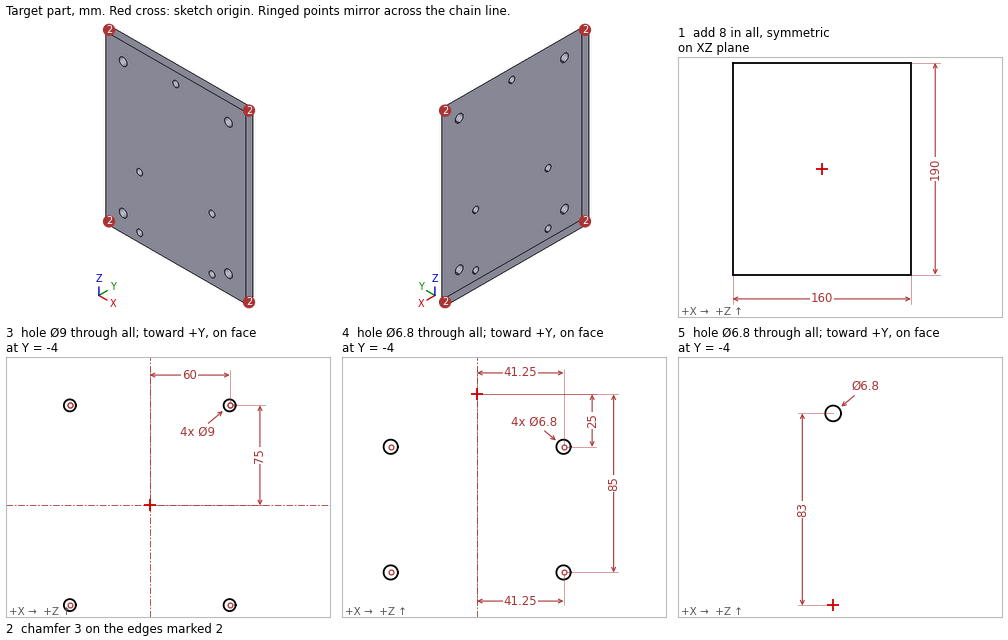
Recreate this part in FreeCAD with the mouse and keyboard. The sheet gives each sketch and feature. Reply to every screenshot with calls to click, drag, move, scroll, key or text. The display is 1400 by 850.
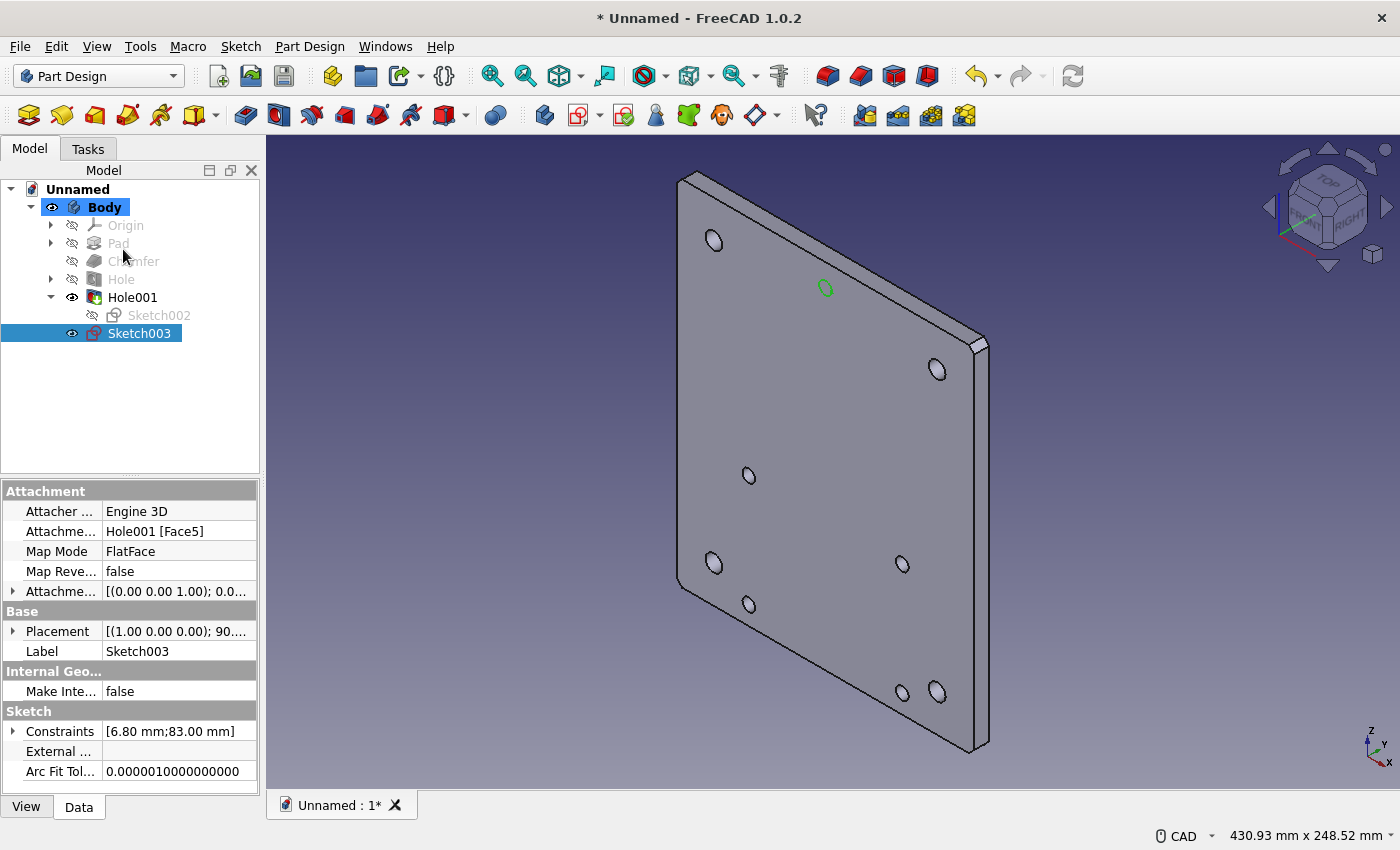
click(279, 116)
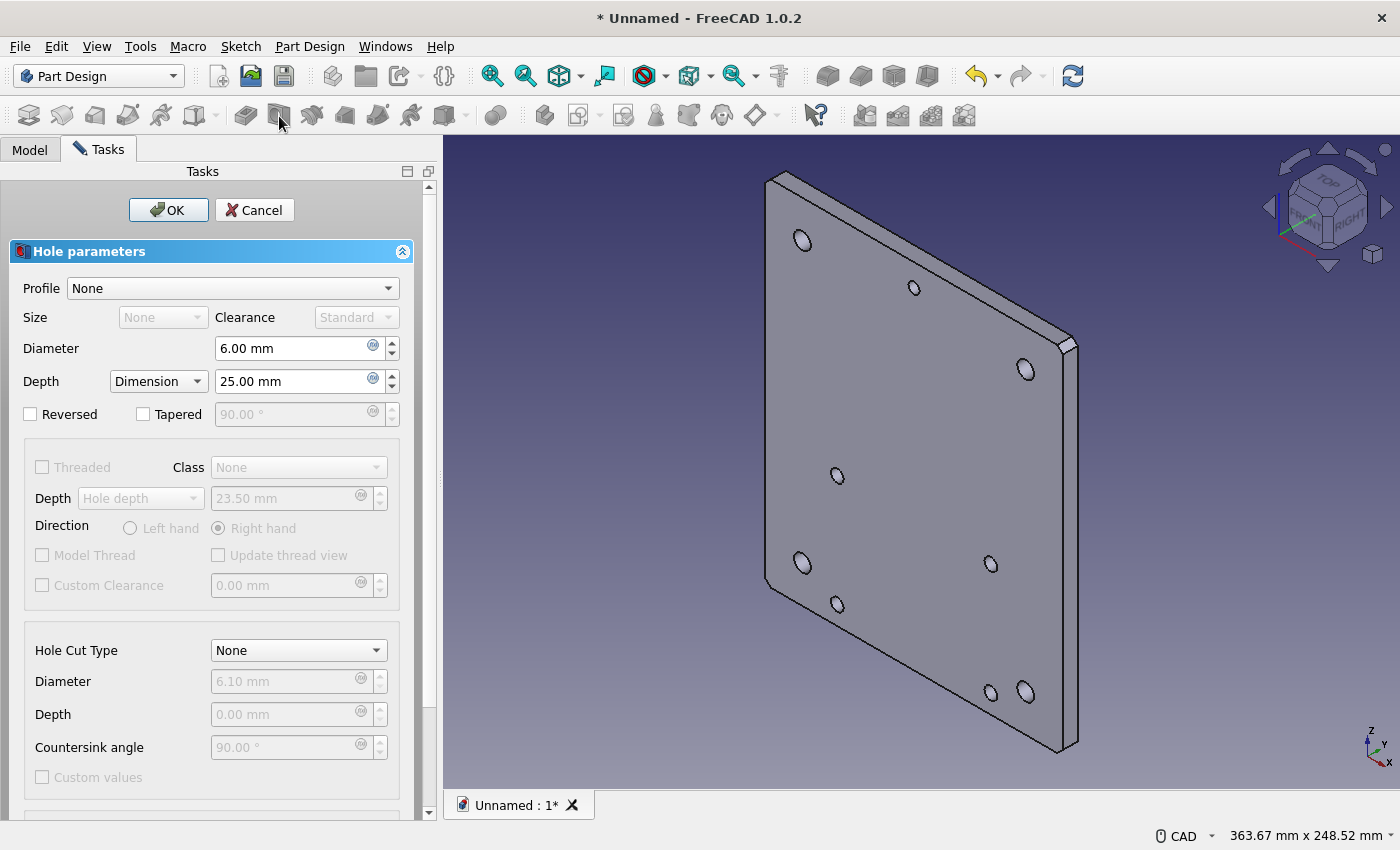
triple_click(300, 348)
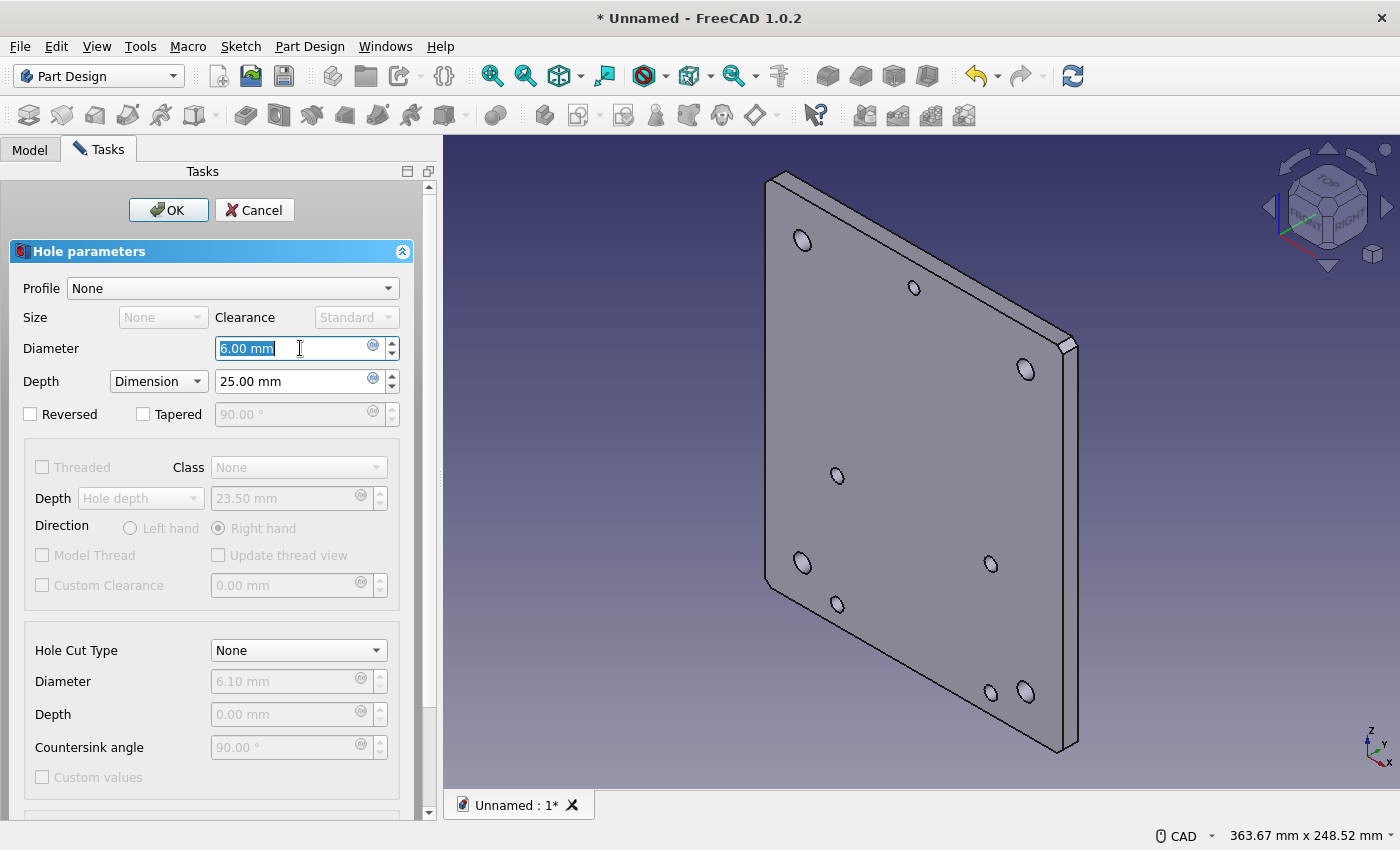
text(6.8)
key(Tab)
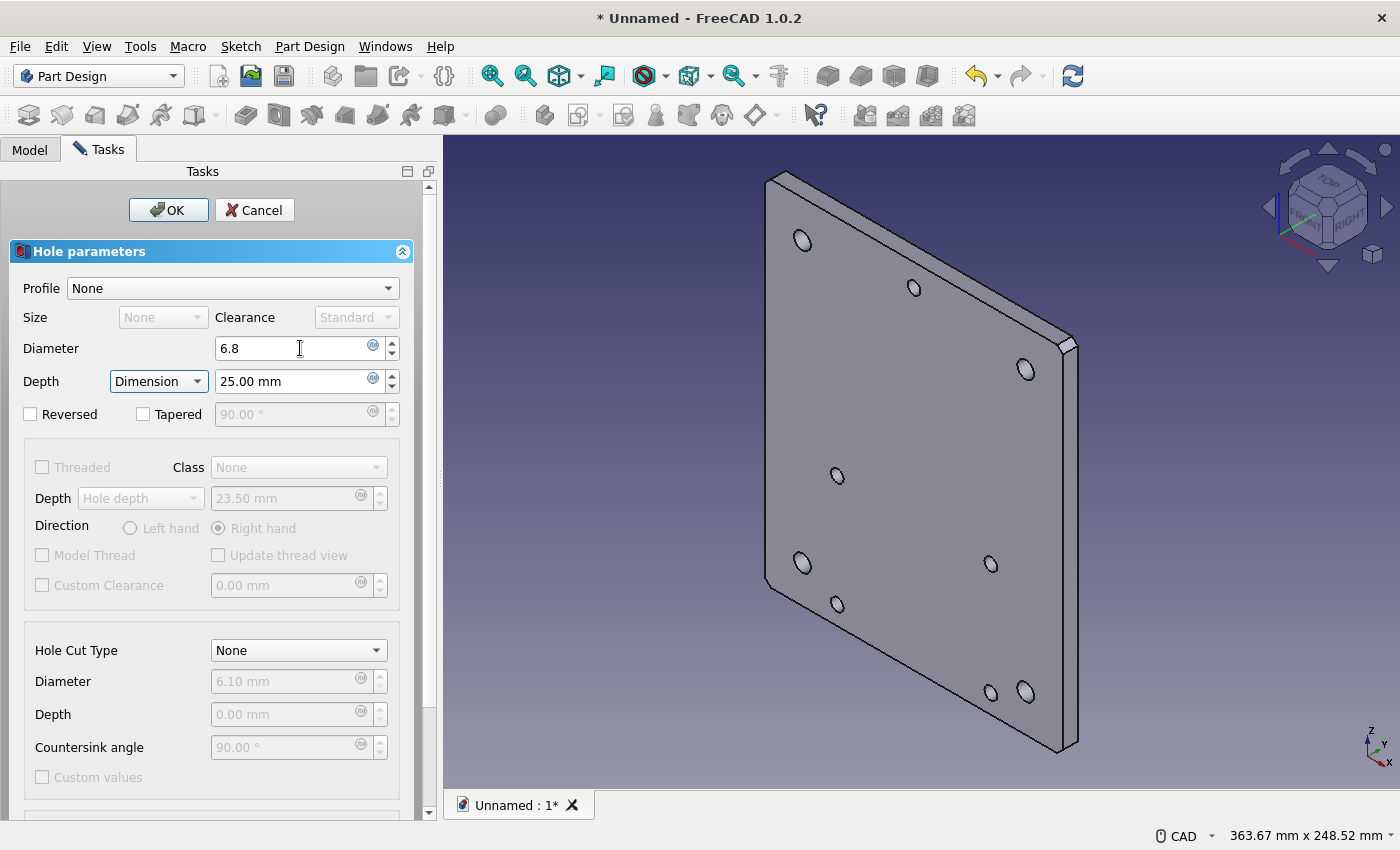
click(160, 382)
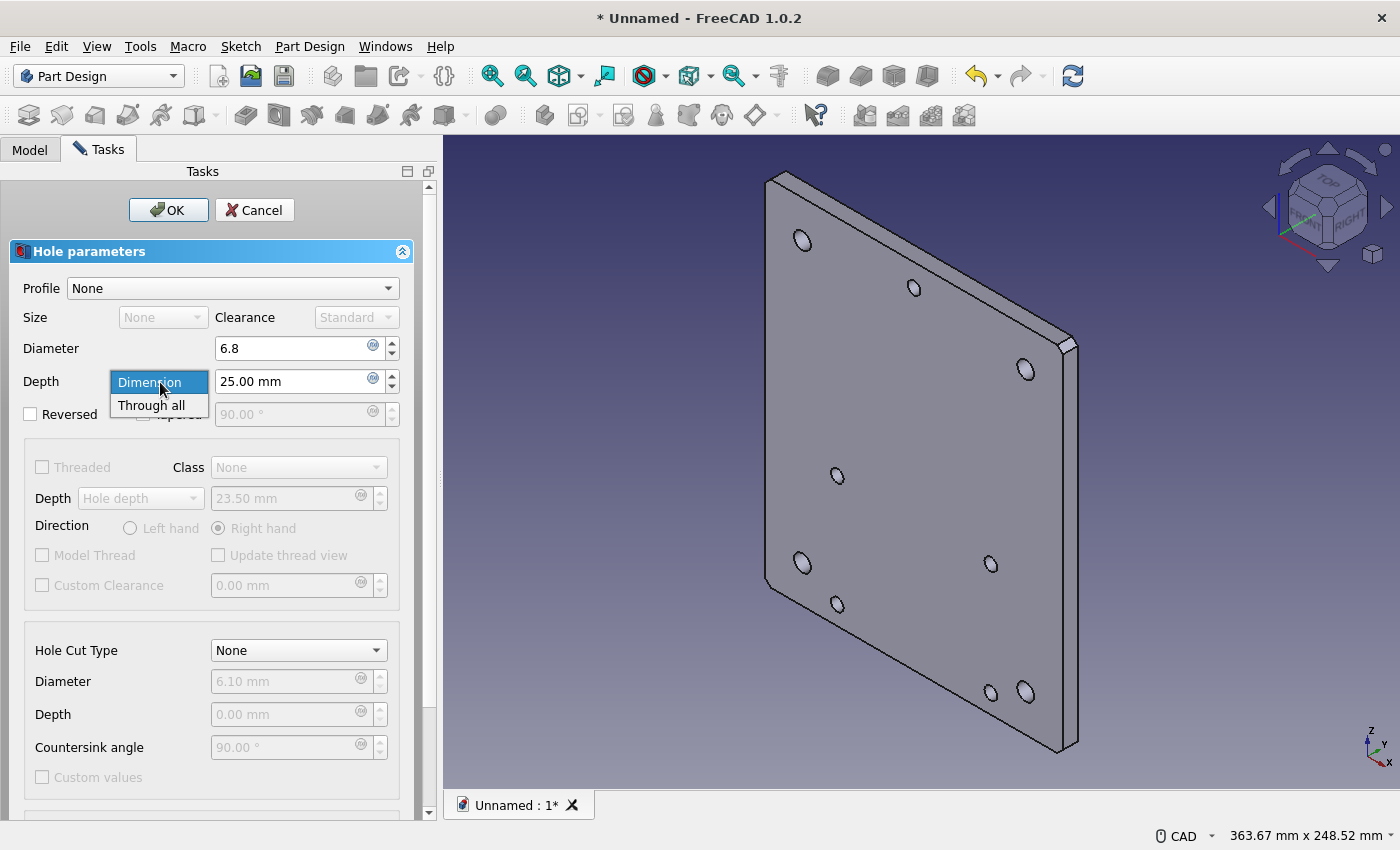
click(158, 406)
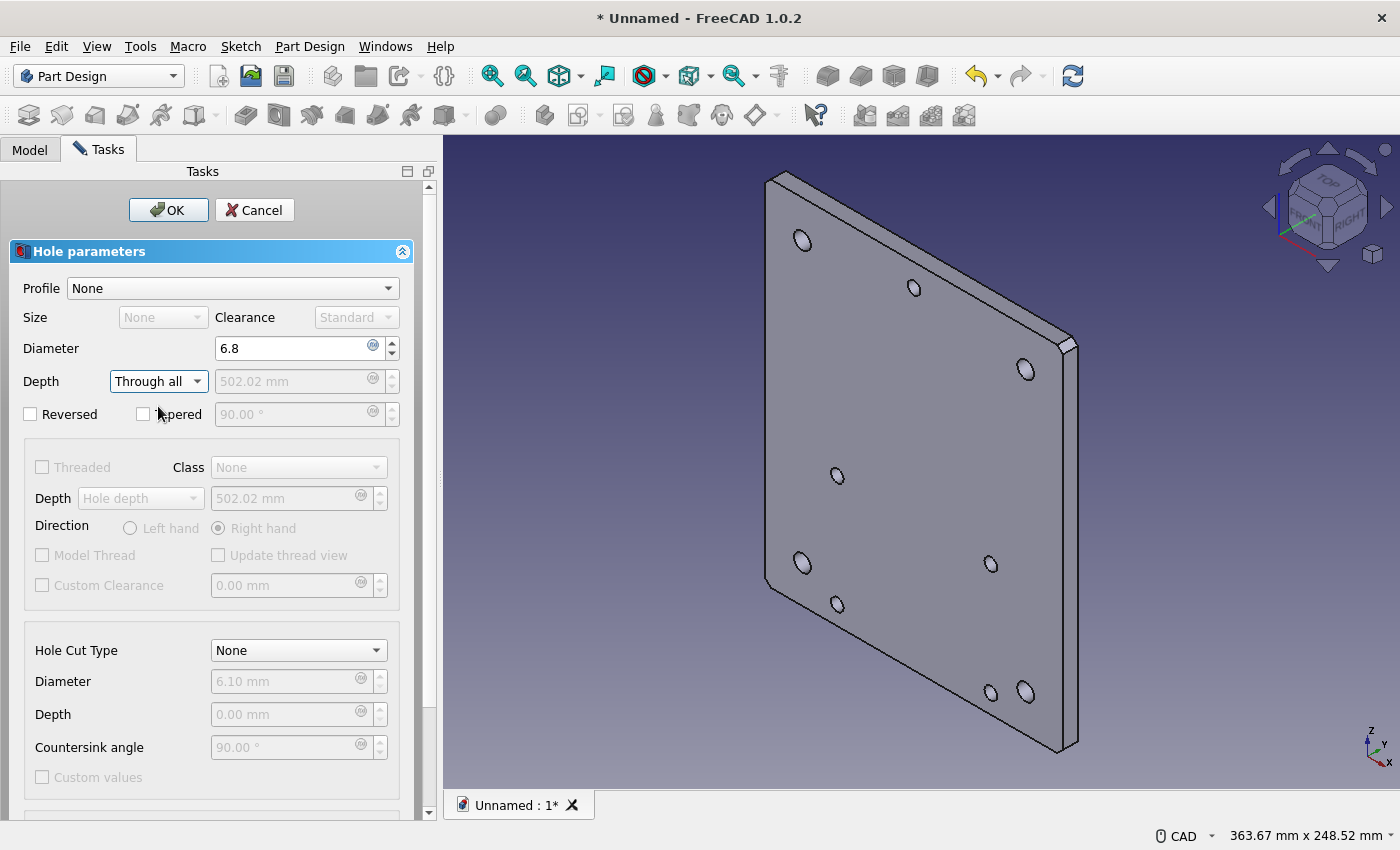
click(169, 210)